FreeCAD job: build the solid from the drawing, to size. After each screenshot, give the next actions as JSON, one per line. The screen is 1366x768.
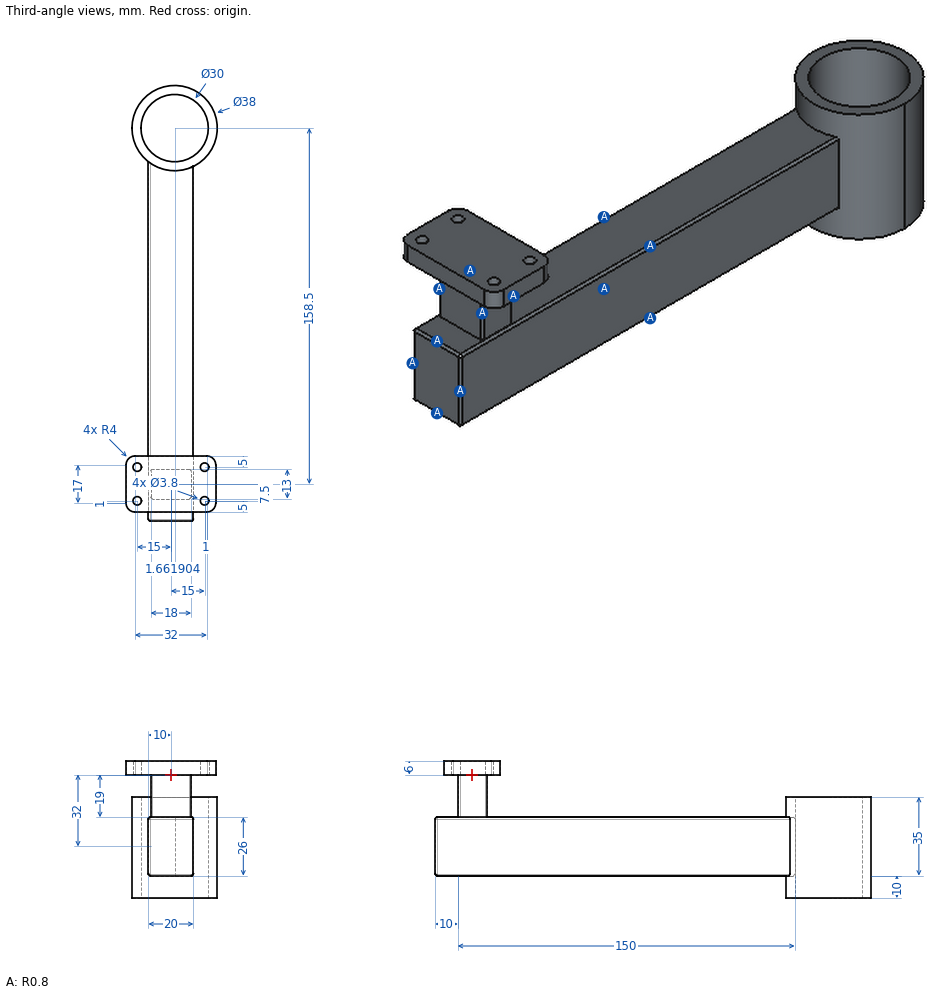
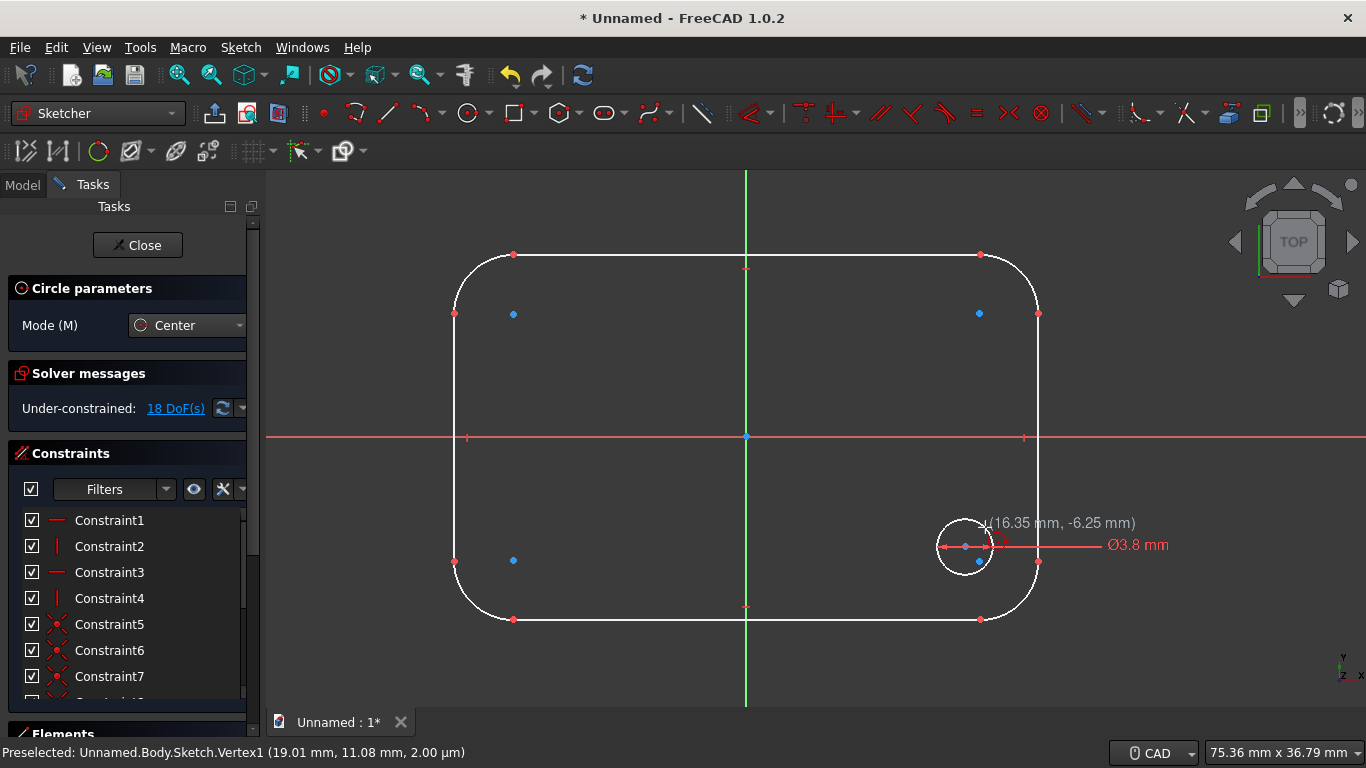
{"action": "left_click", "coordinate": [527, 546]}
{"action": "mouse_move", "coordinate": [547, 527]}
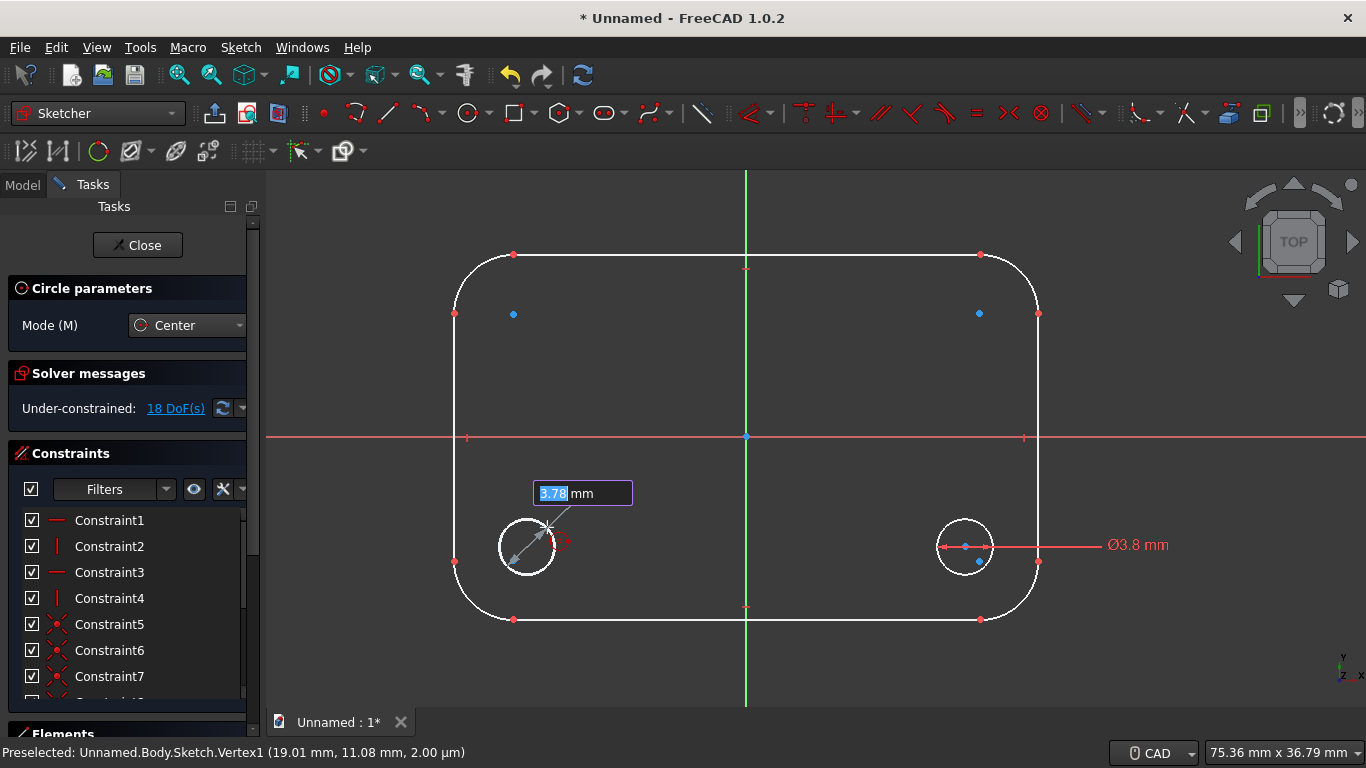
{"action": "type", "text": "3.8"}
{"action": "key", "text": "Return"}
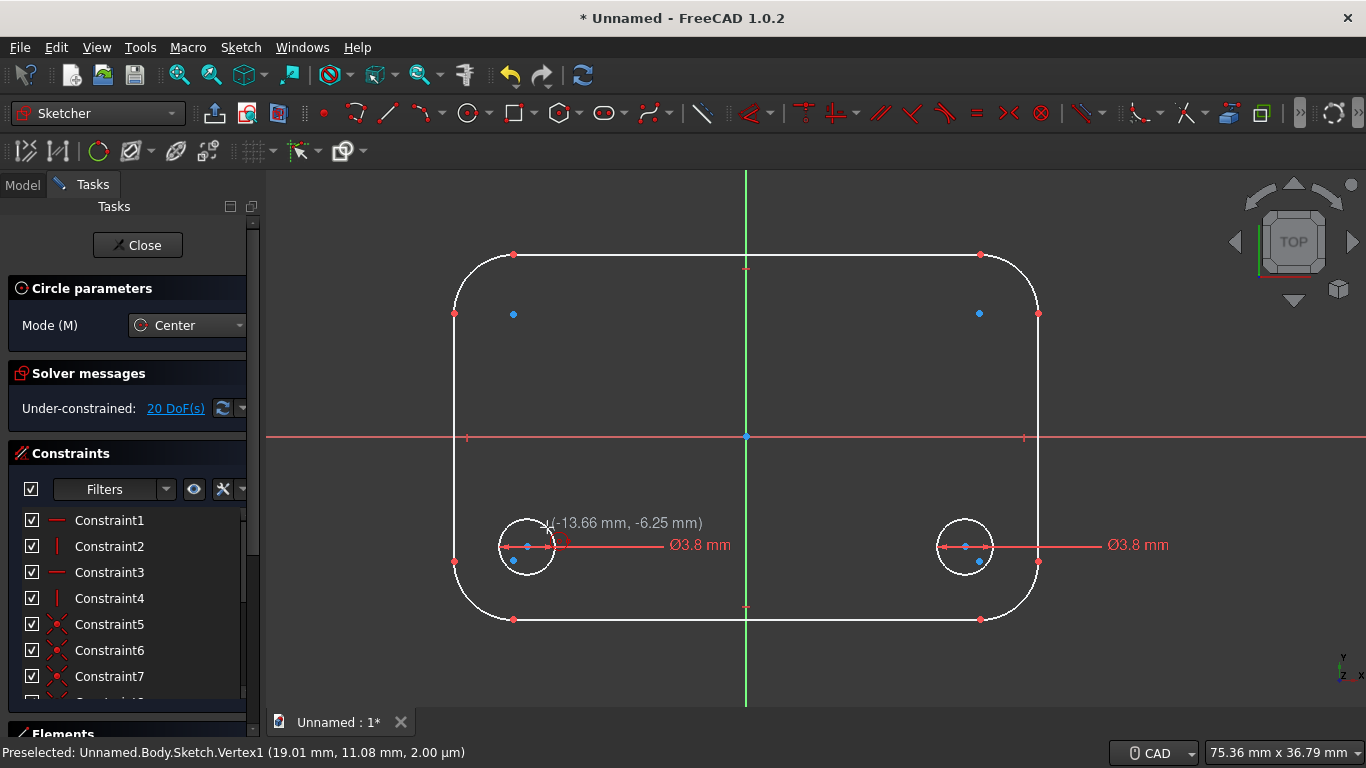
{"action": "left_click", "coordinate": [965, 327]}
{"action": "mouse_move", "coordinate": [946, 308]}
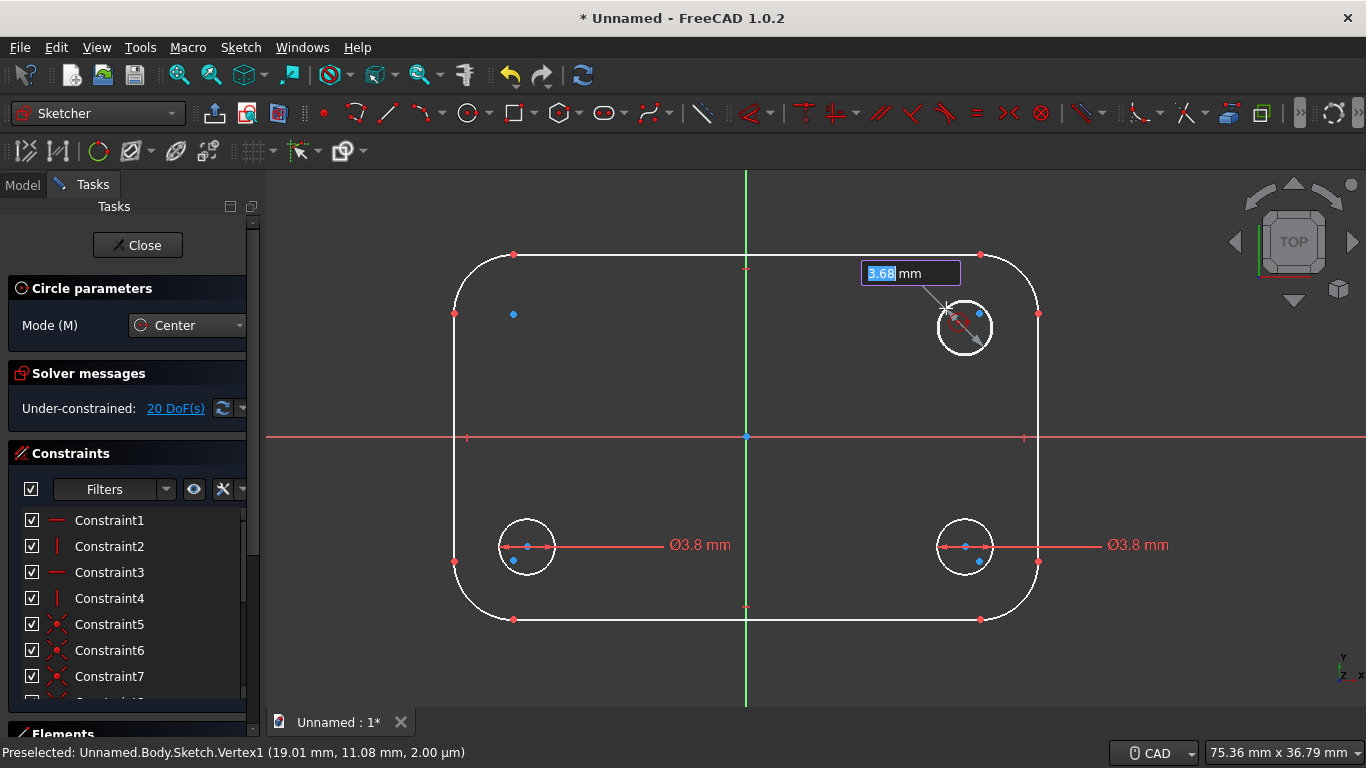
{"action": "type", "text": "3.8"}
{"action": "key", "text": "Return"}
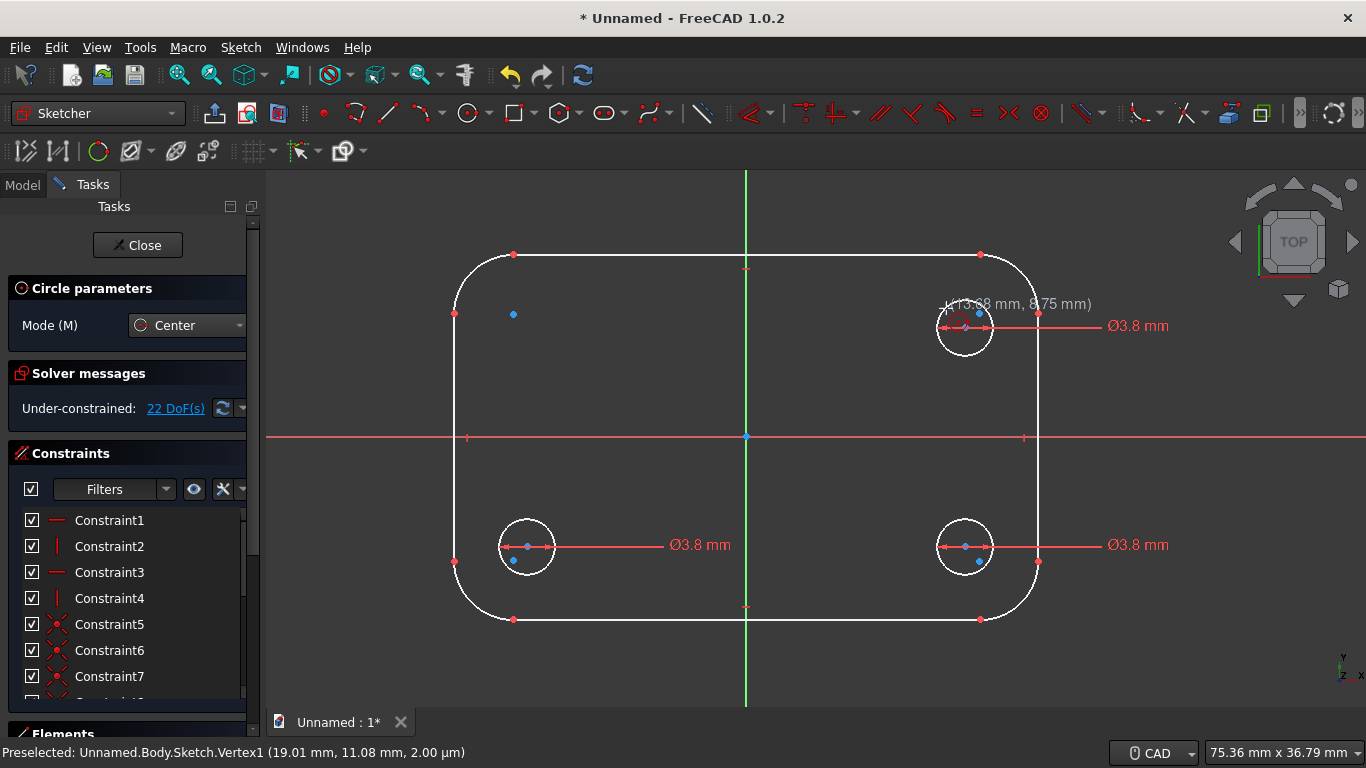
{"action": "left_click", "coordinate": [527, 327]}
{"action": "mouse_move", "coordinate": [547, 308]}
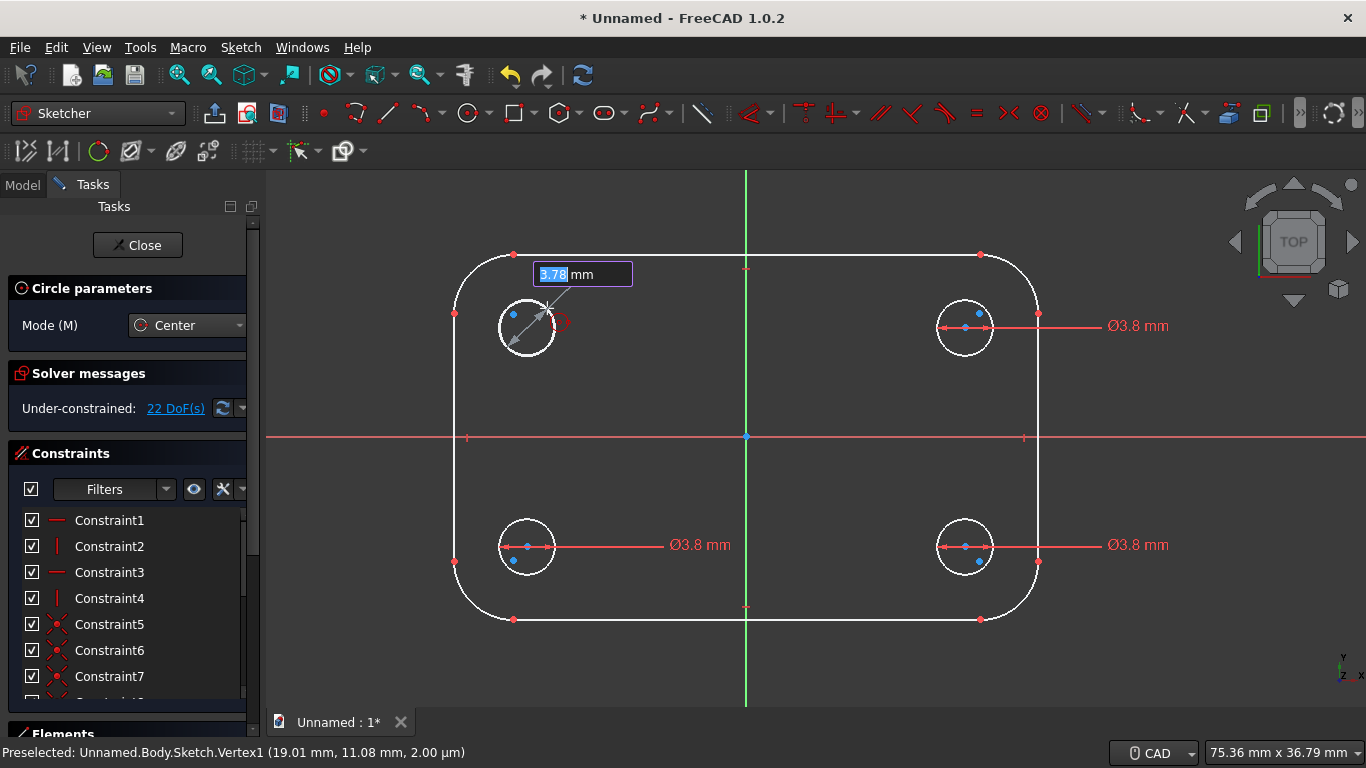
{"action": "type", "text": "3.8"}
{"action": "key", "text": "Return"}
{"action": "key", "text": "Escape"}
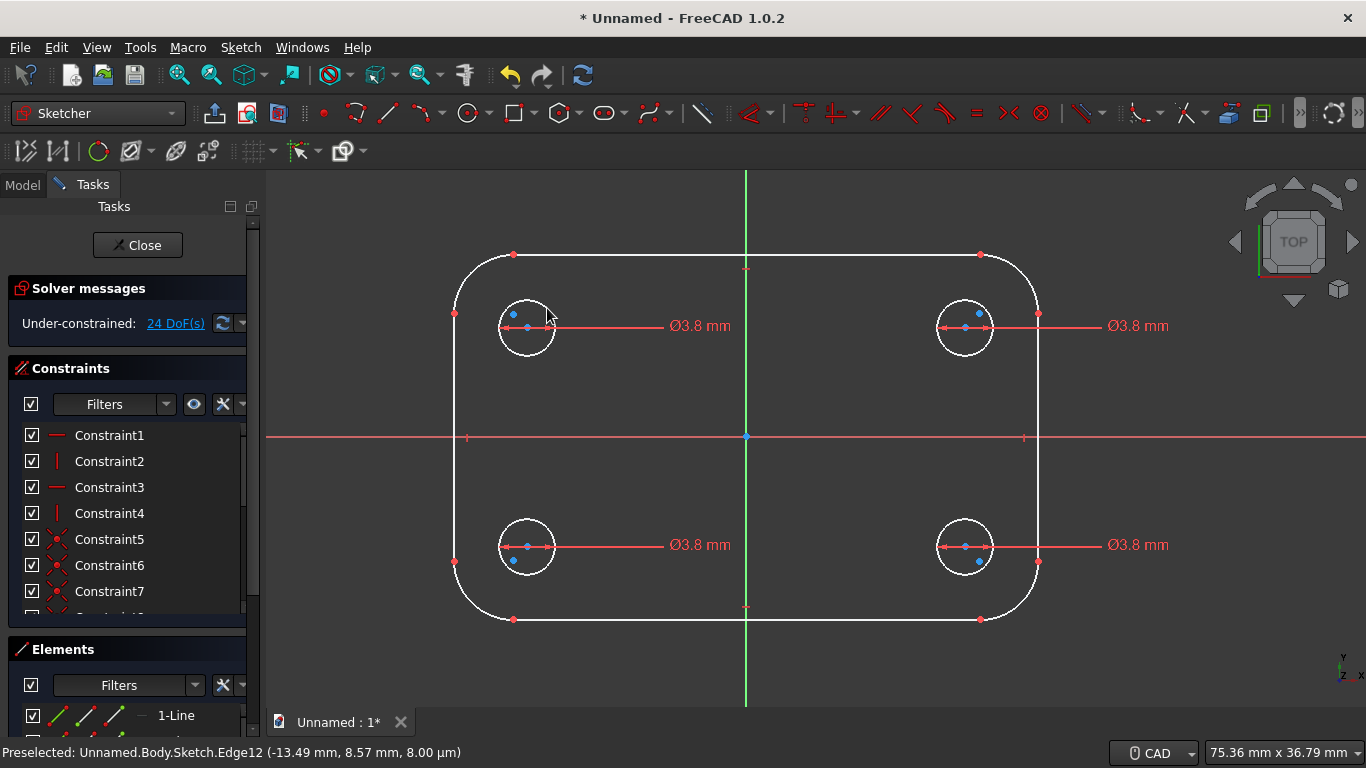
{"action": "left_click", "coordinate": [840, 255]}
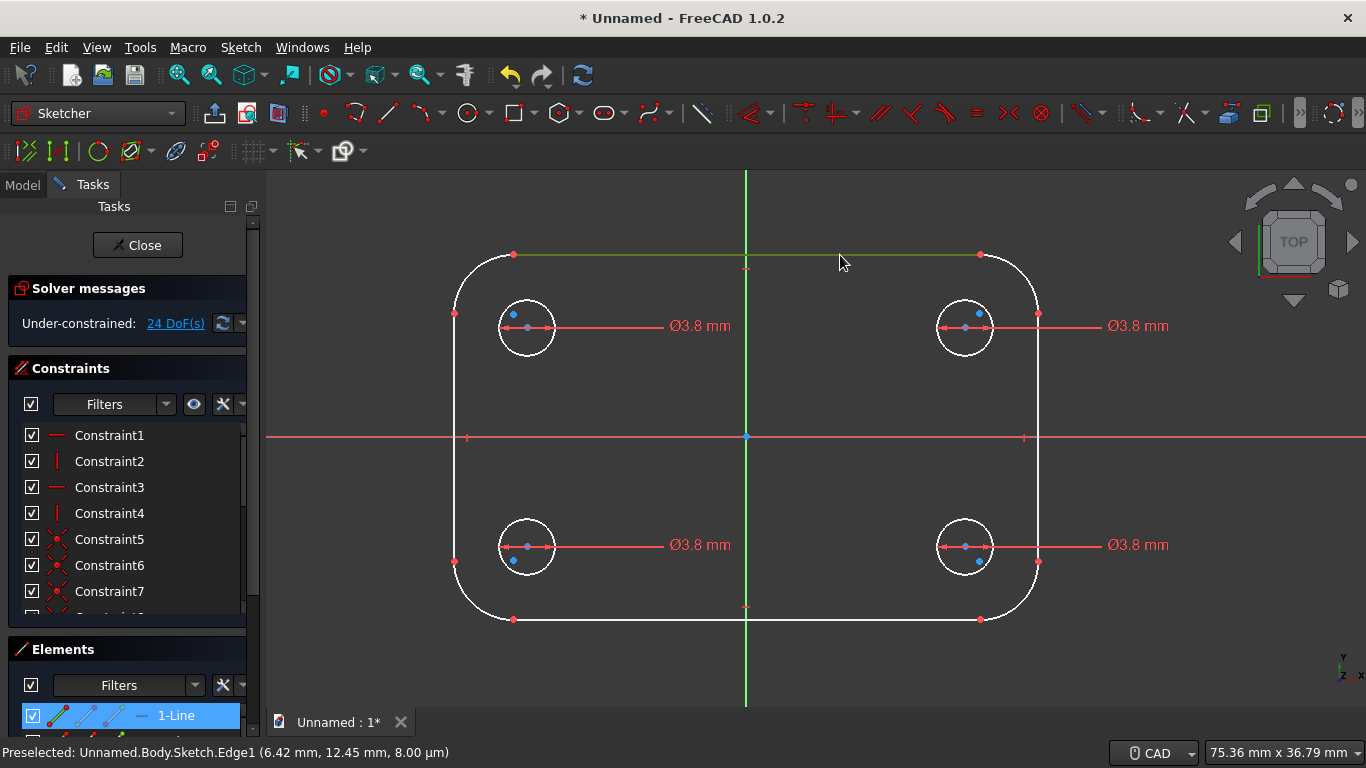
{"action": "left_click", "coordinate": [486, 262]}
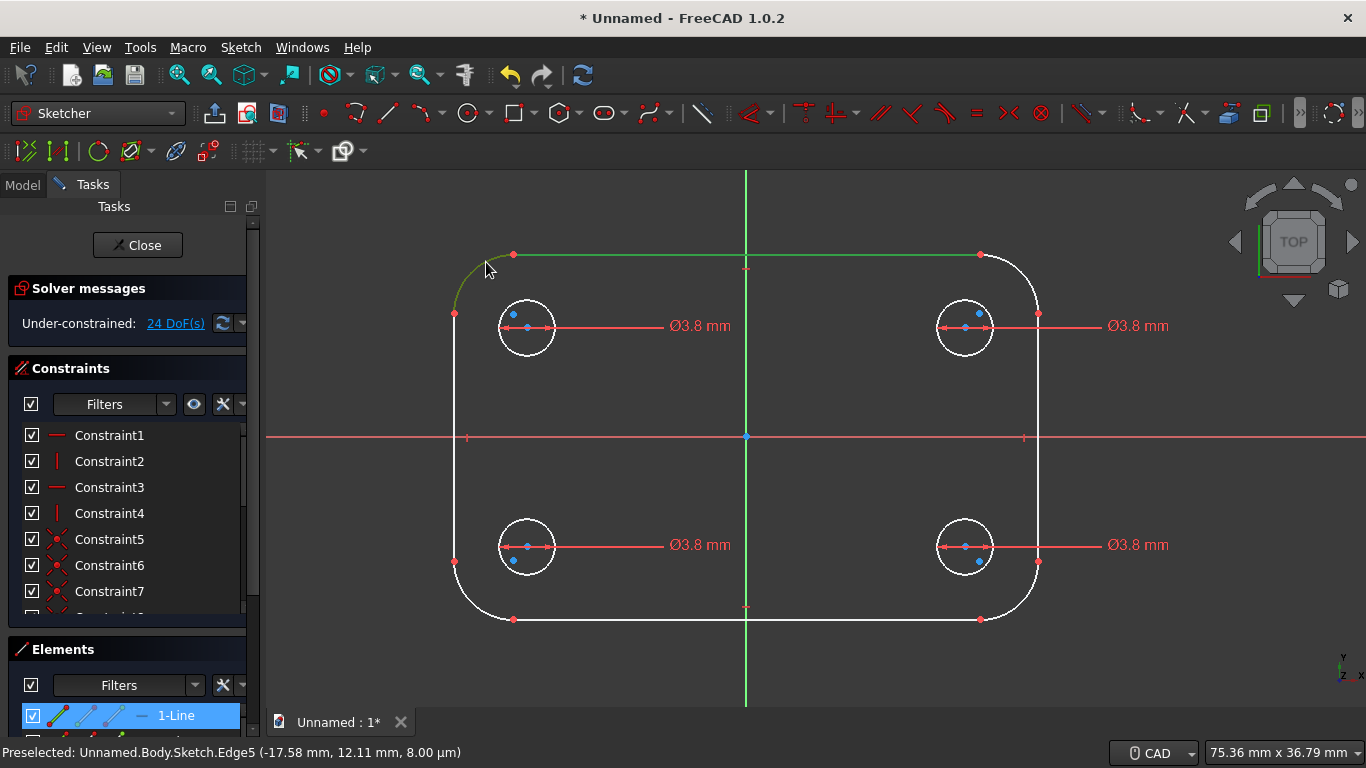
{"action": "left_click", "coordinate": [946, 114]}